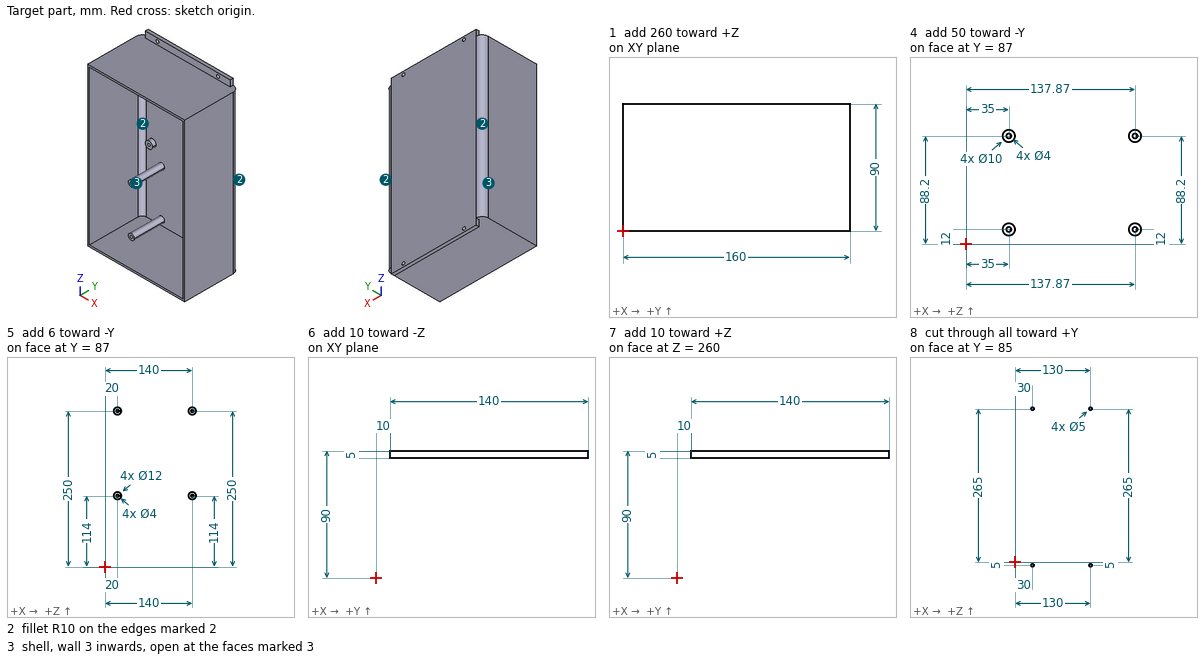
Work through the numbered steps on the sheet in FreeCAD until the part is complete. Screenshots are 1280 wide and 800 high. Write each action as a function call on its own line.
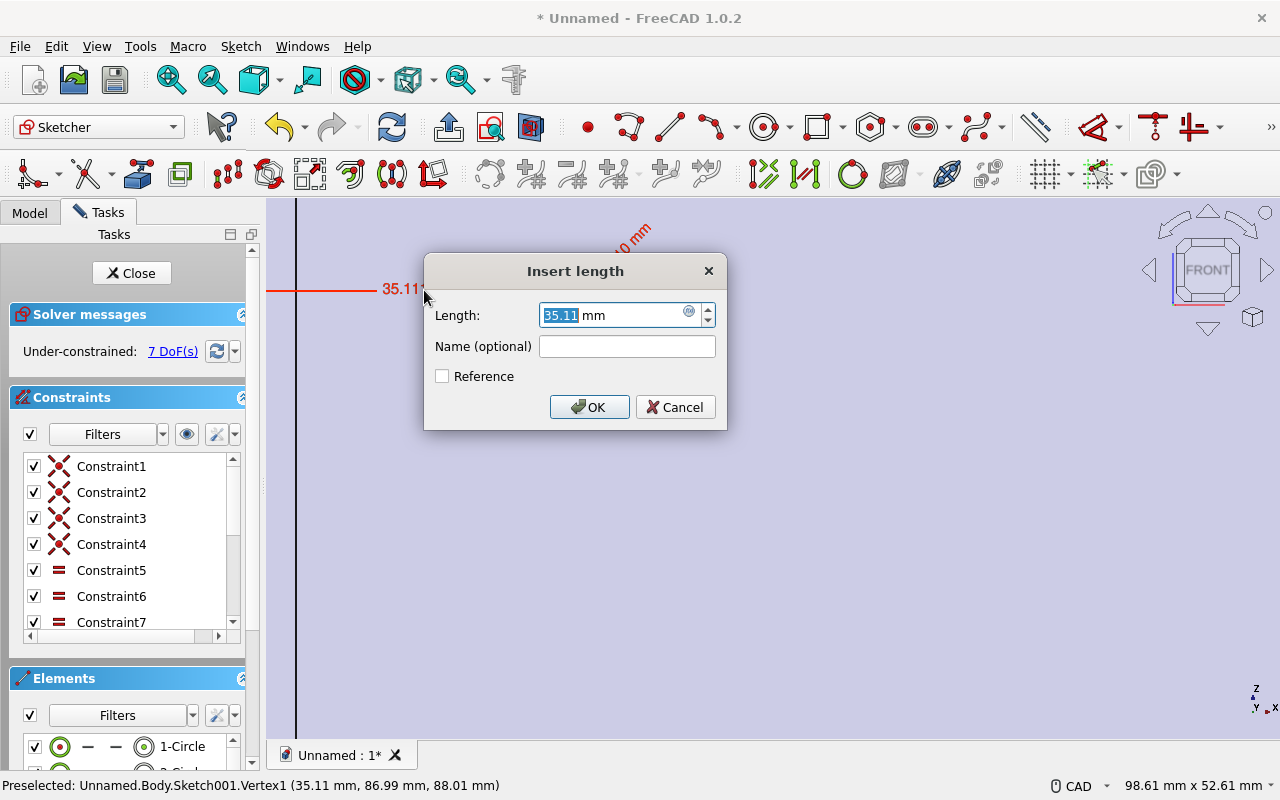
text(35)
key(Return)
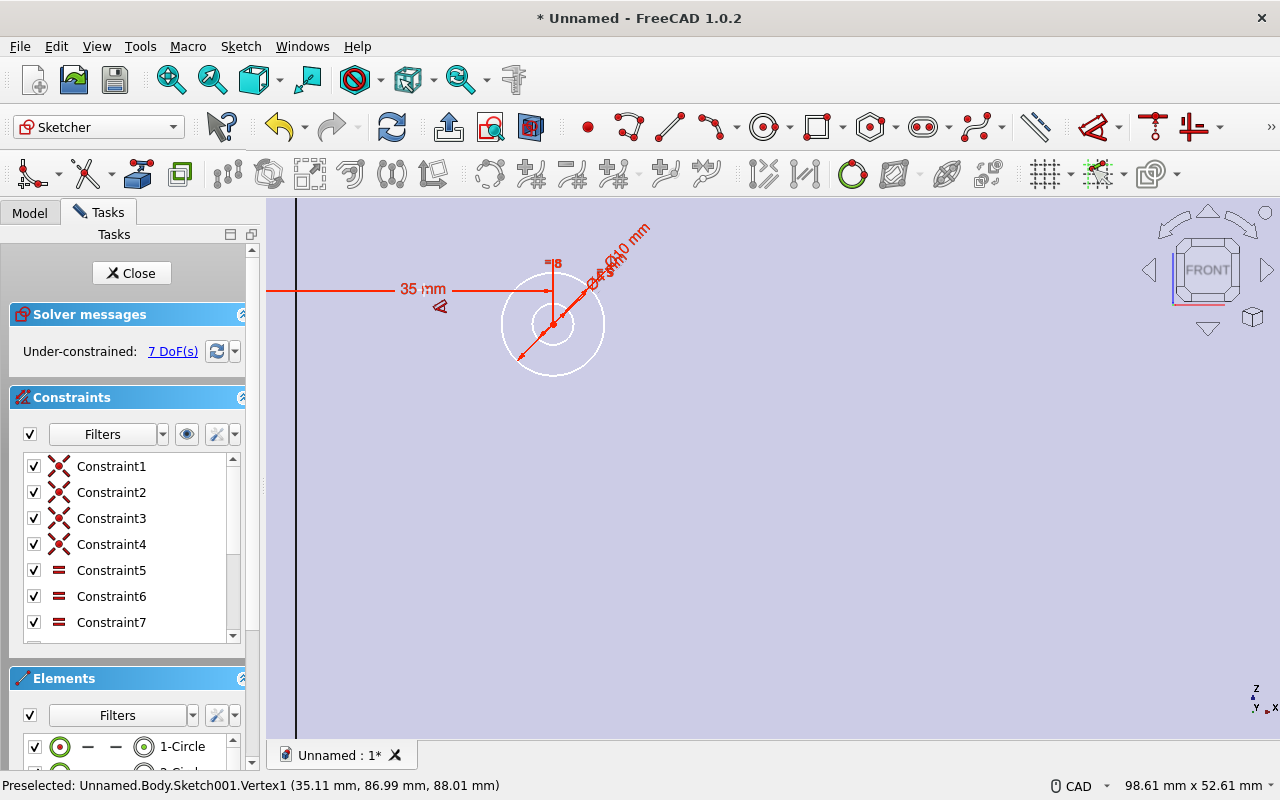
scroll(575, 305, down, 5)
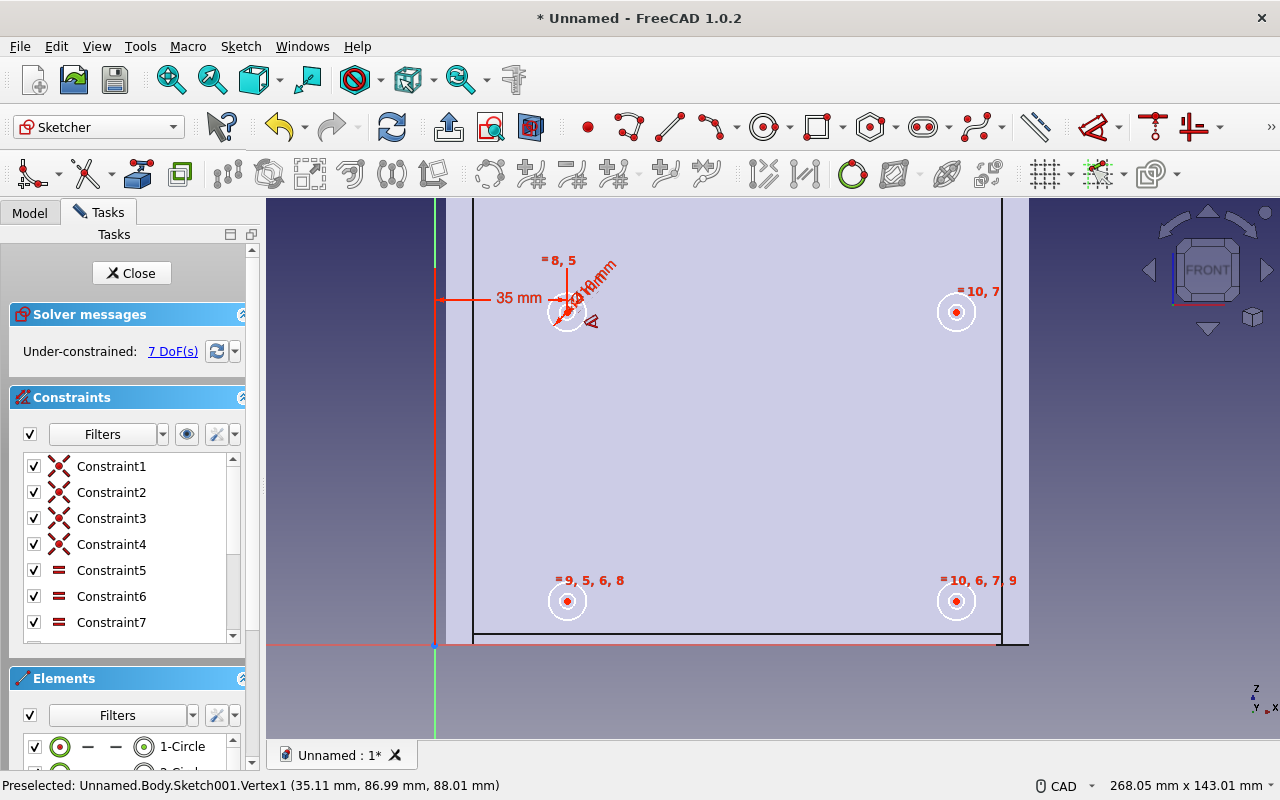
click(568, 601)
click(501, 679)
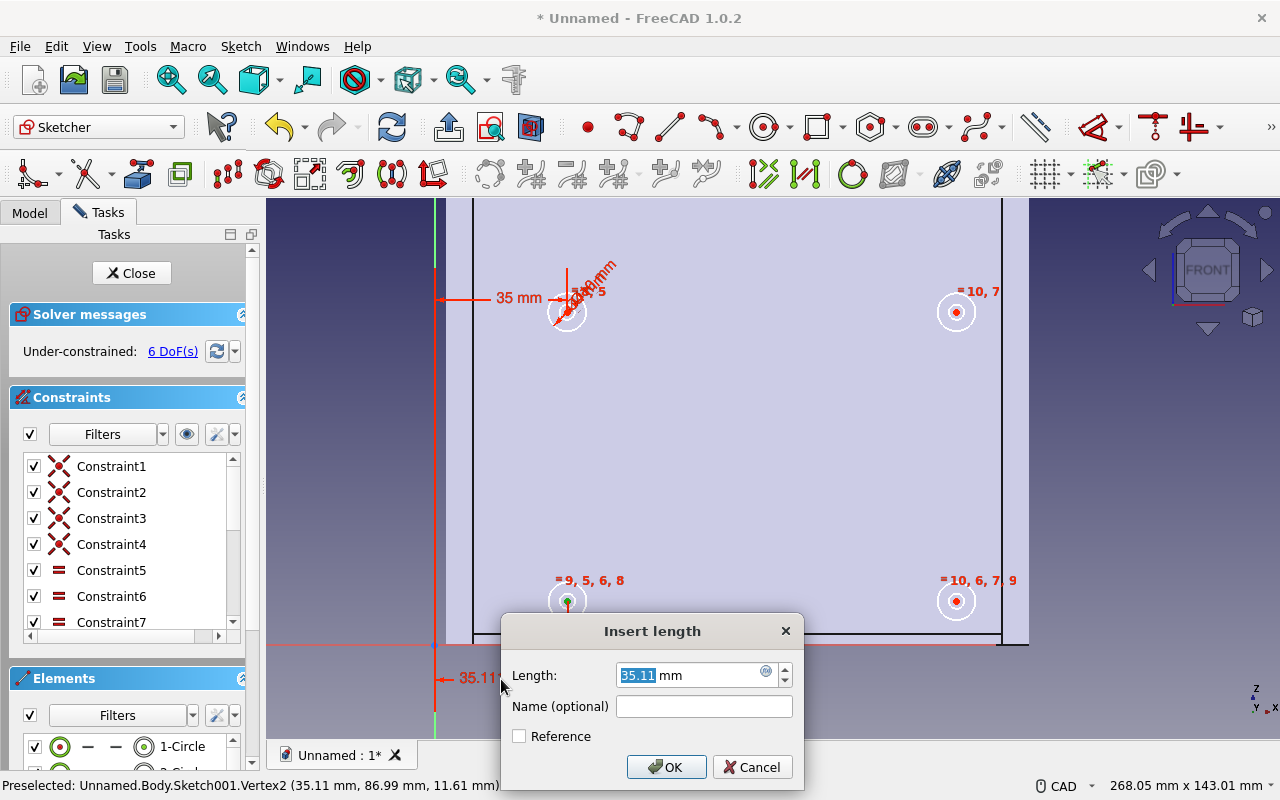
text(35)
key(Return)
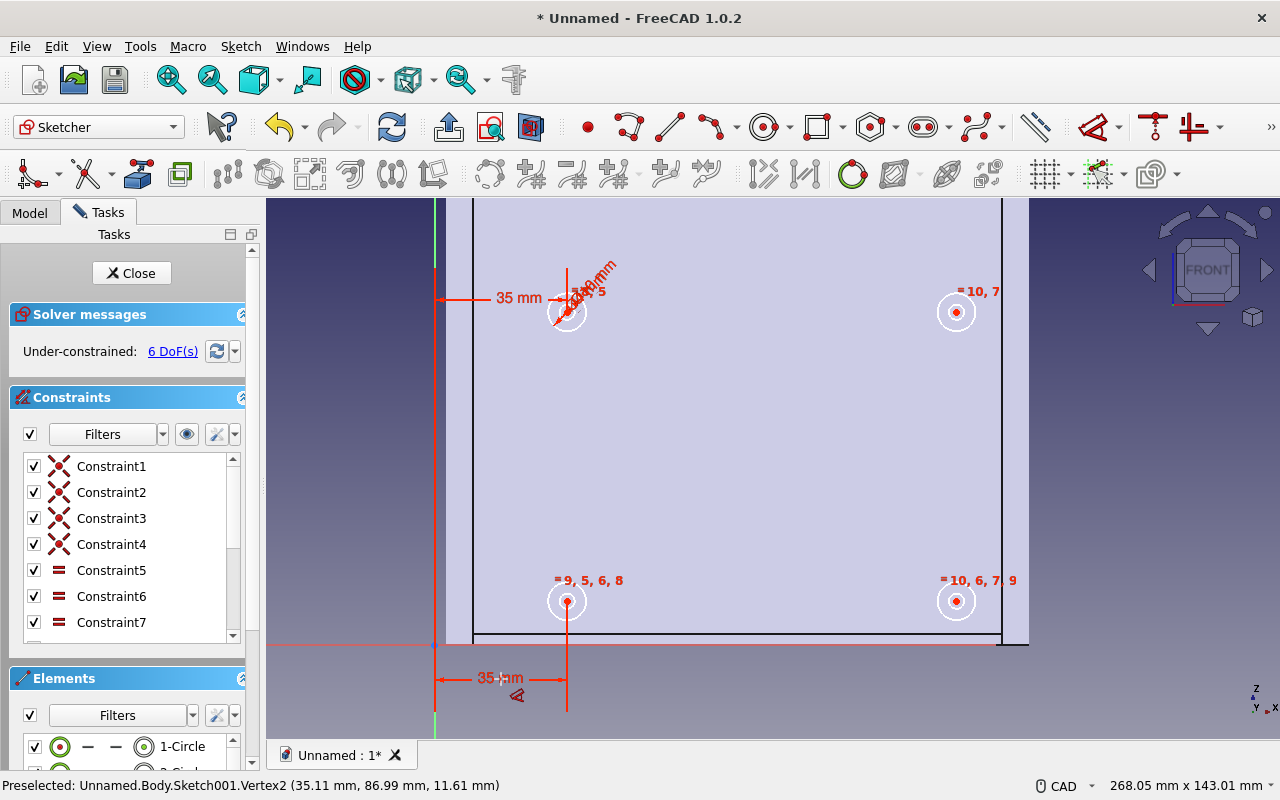
click(567, 601)
click(401, 623)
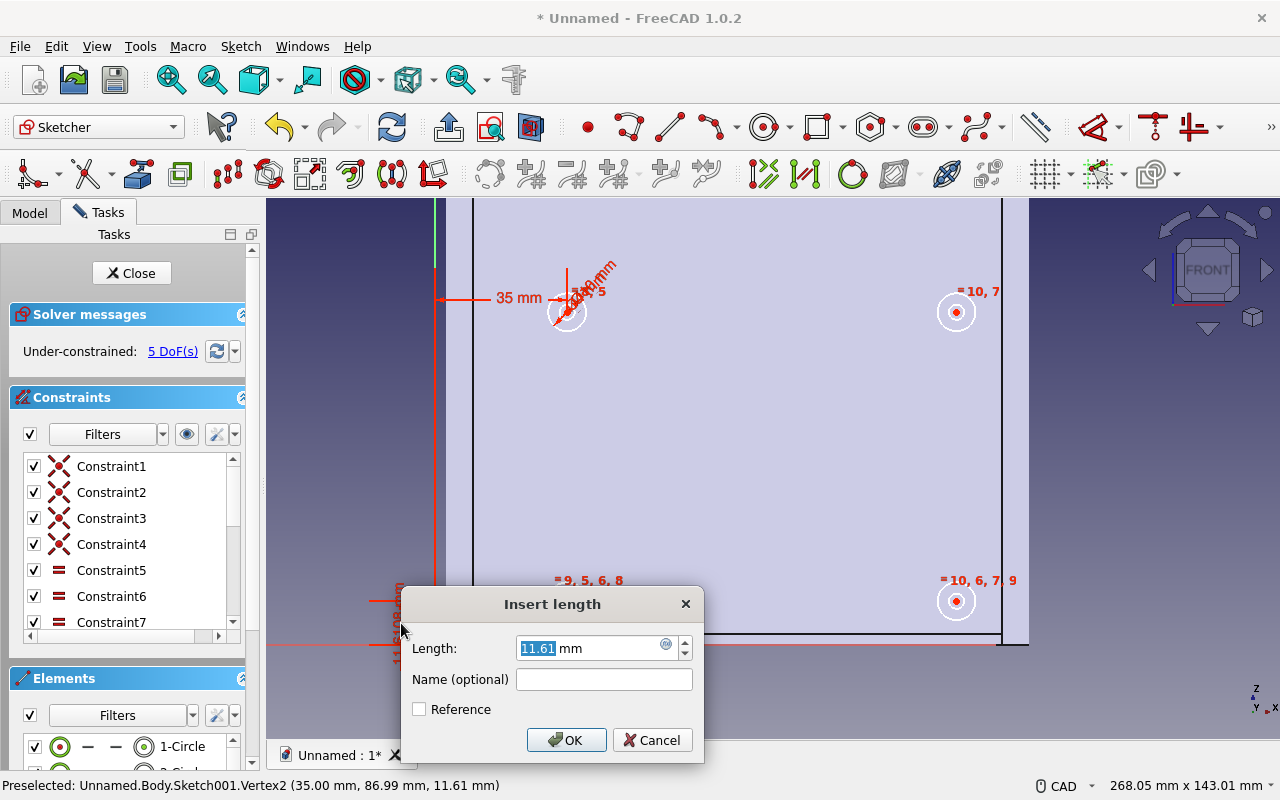
text(12)
key(Return)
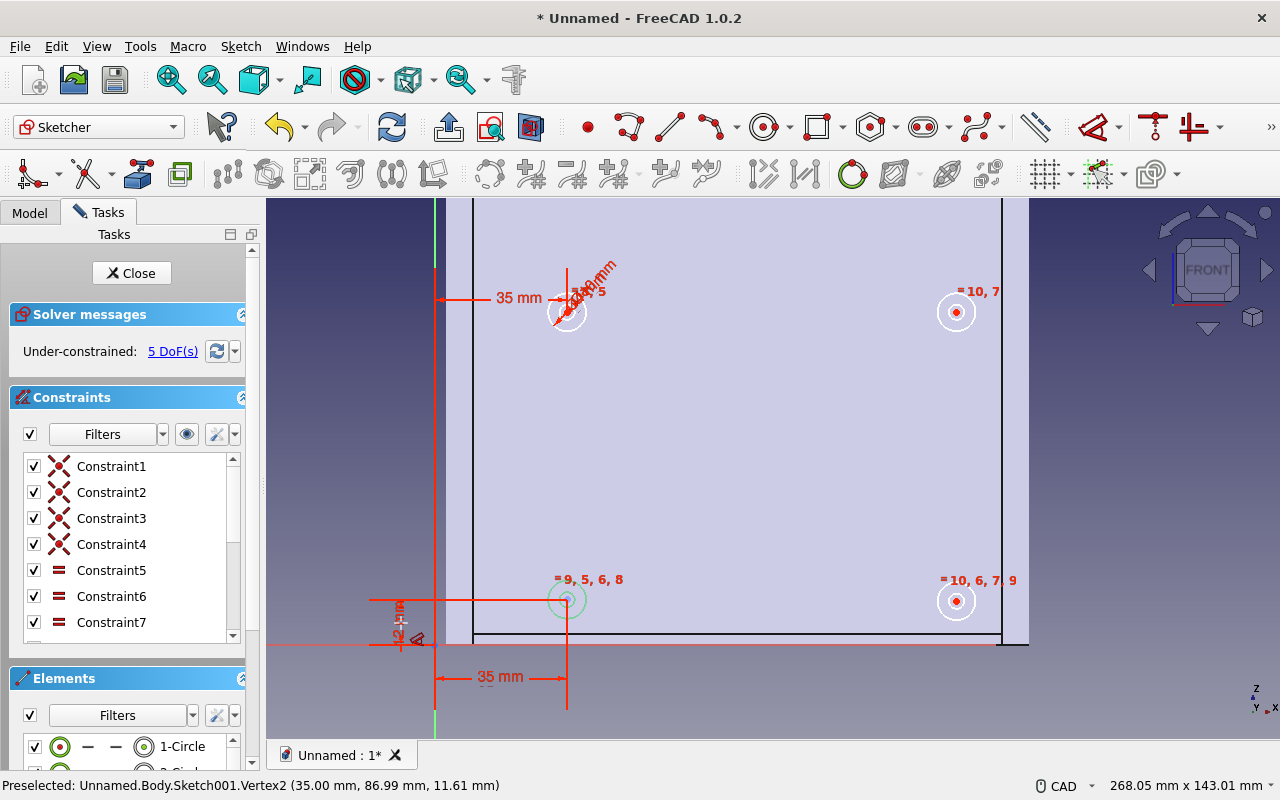
click(957, 601)
click(991, 623)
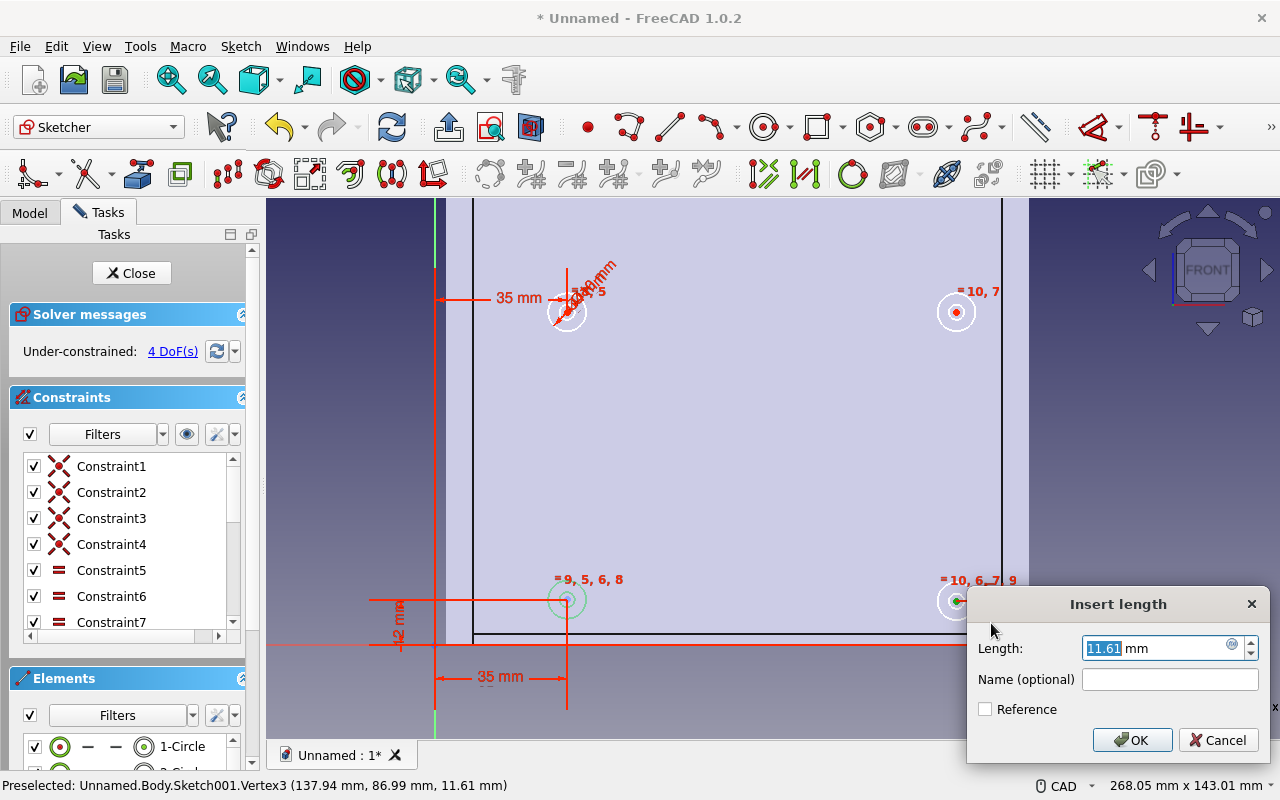
text(12)
key(Return)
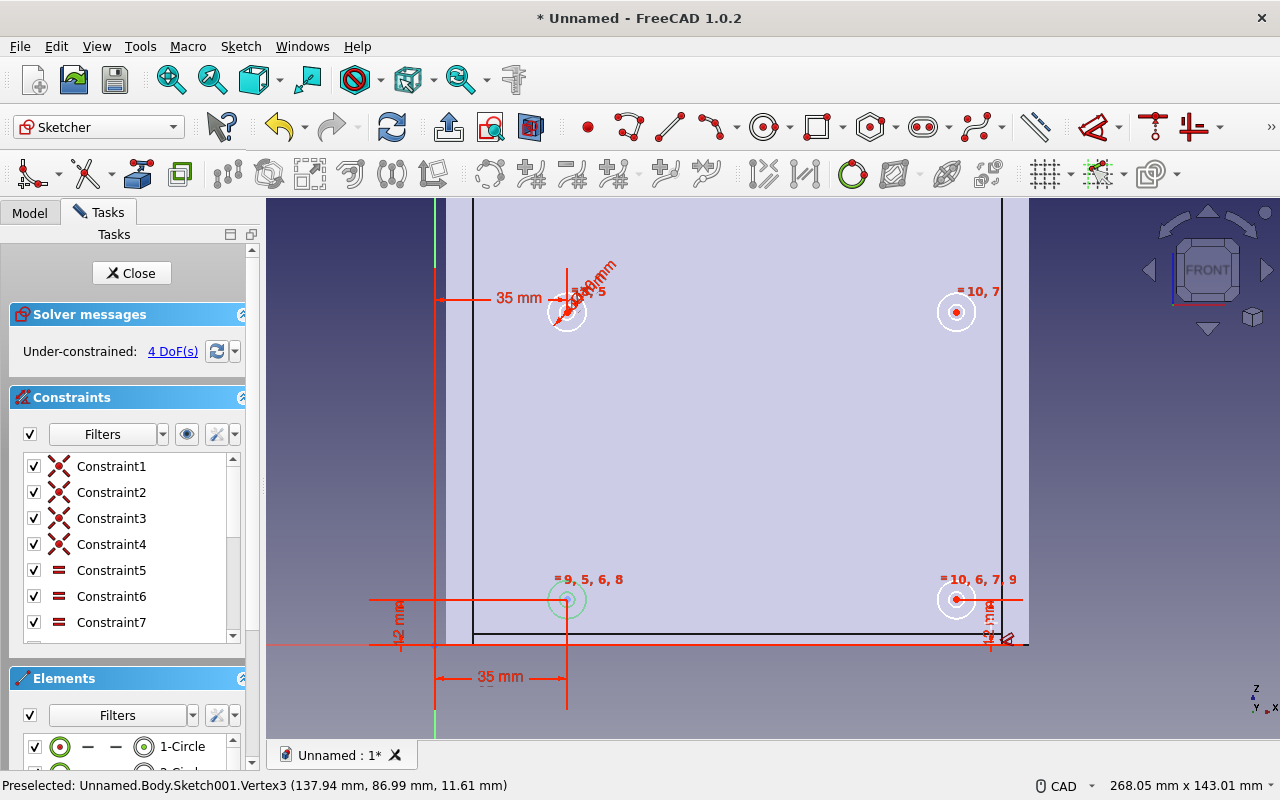
click(567, 312)
click(401, 479)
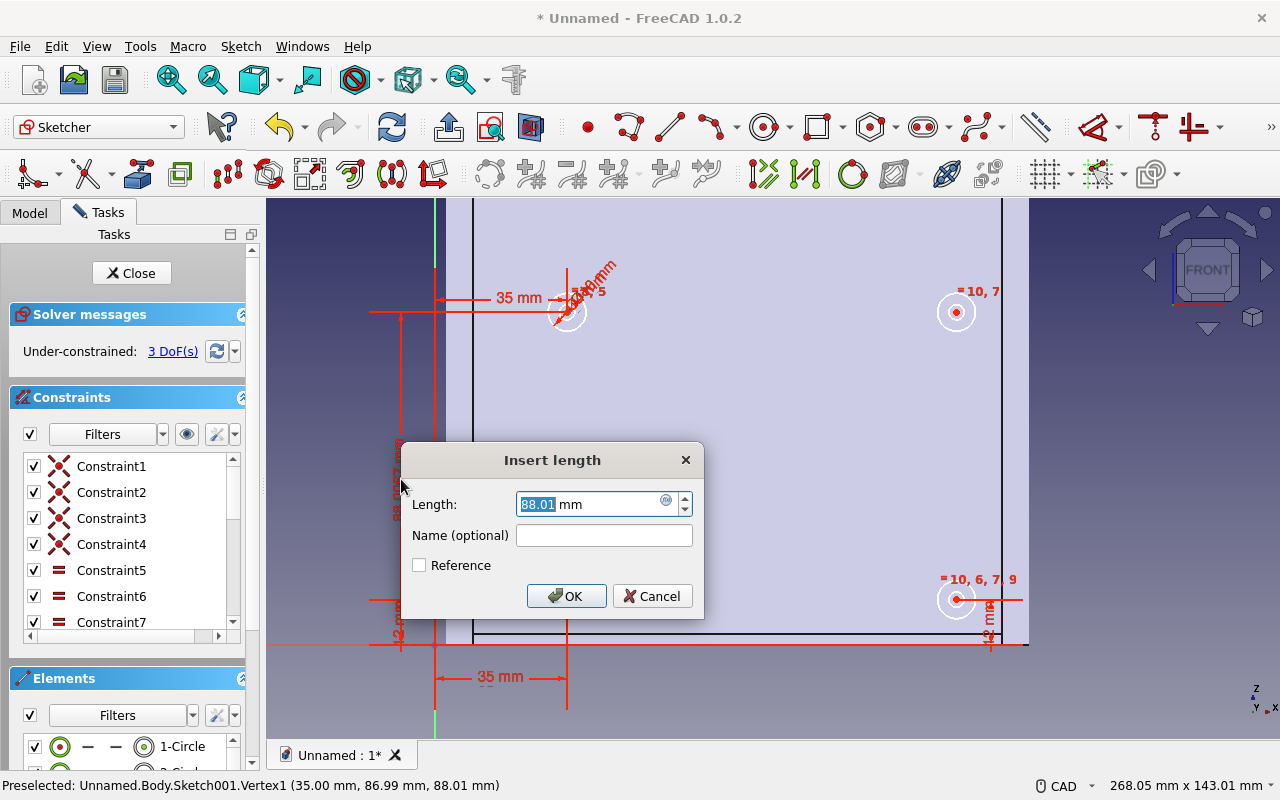
text(88.2)
key(Return)